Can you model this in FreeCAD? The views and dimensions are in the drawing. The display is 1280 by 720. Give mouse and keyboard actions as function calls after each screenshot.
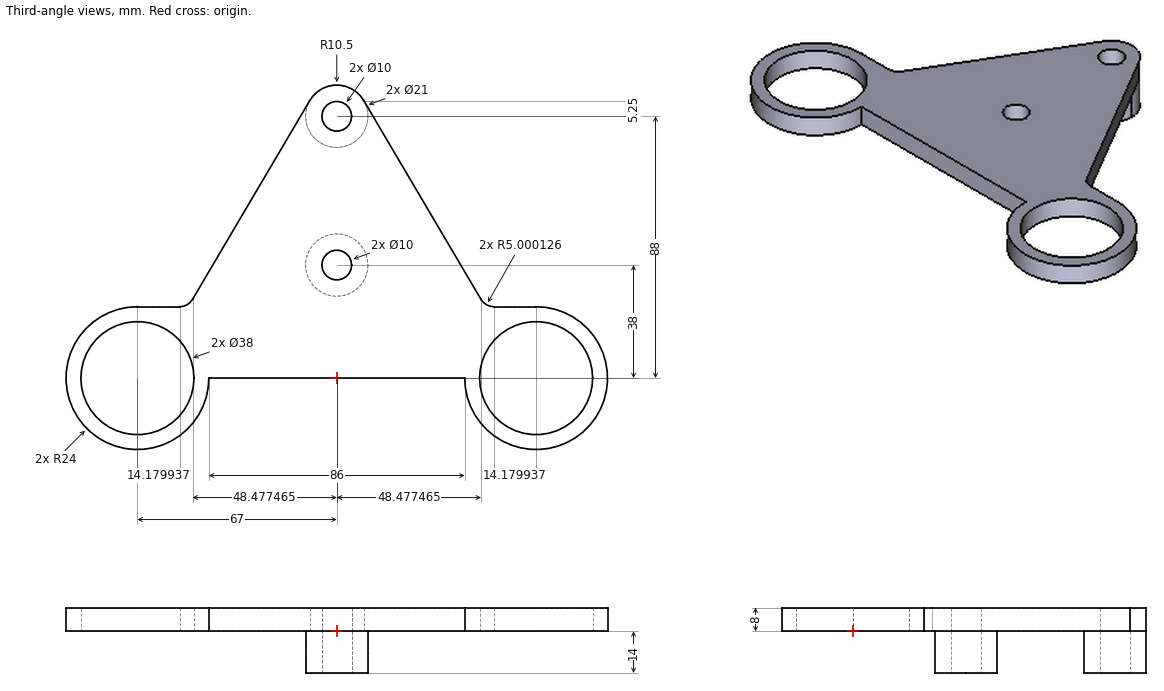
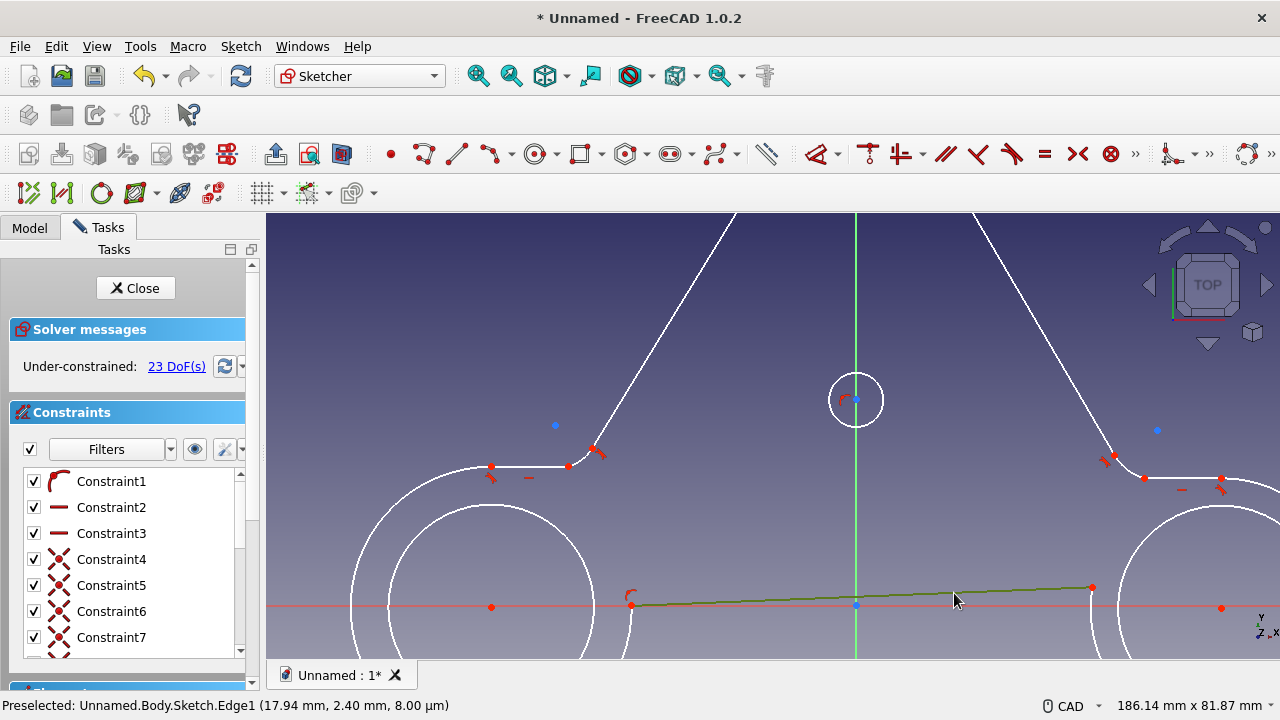
key(h)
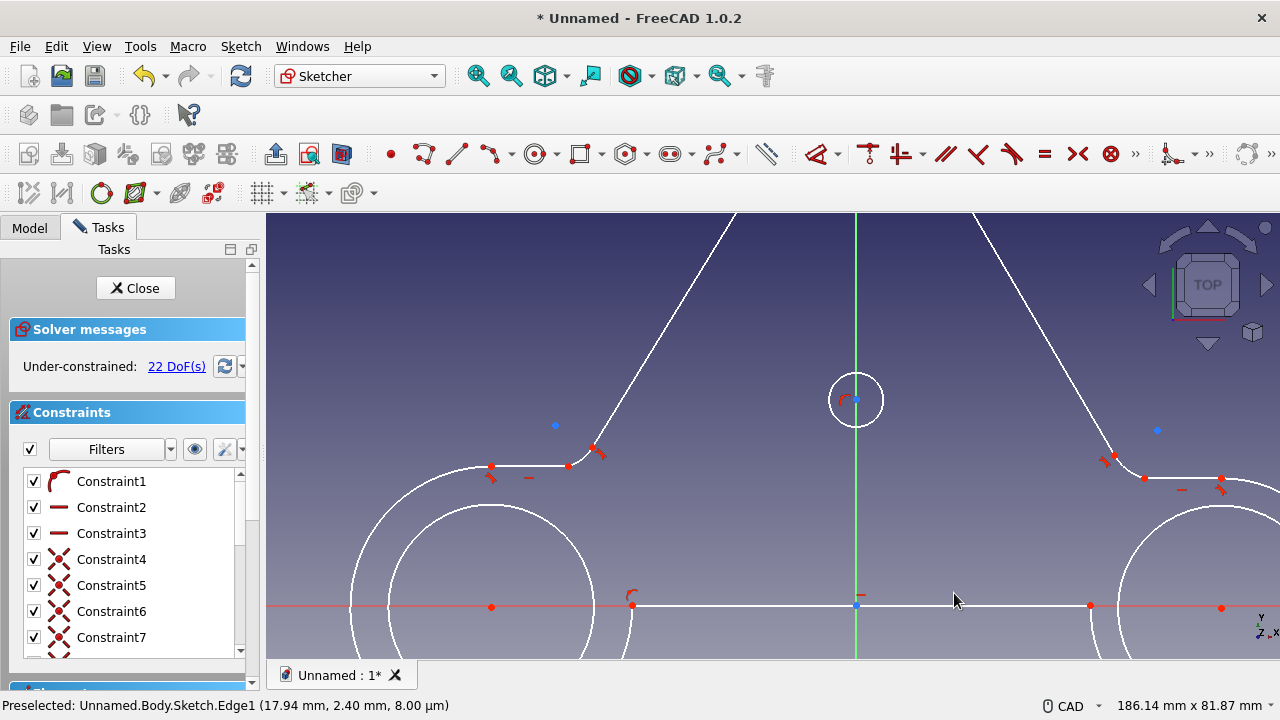
scroll(581, 474, down, 4)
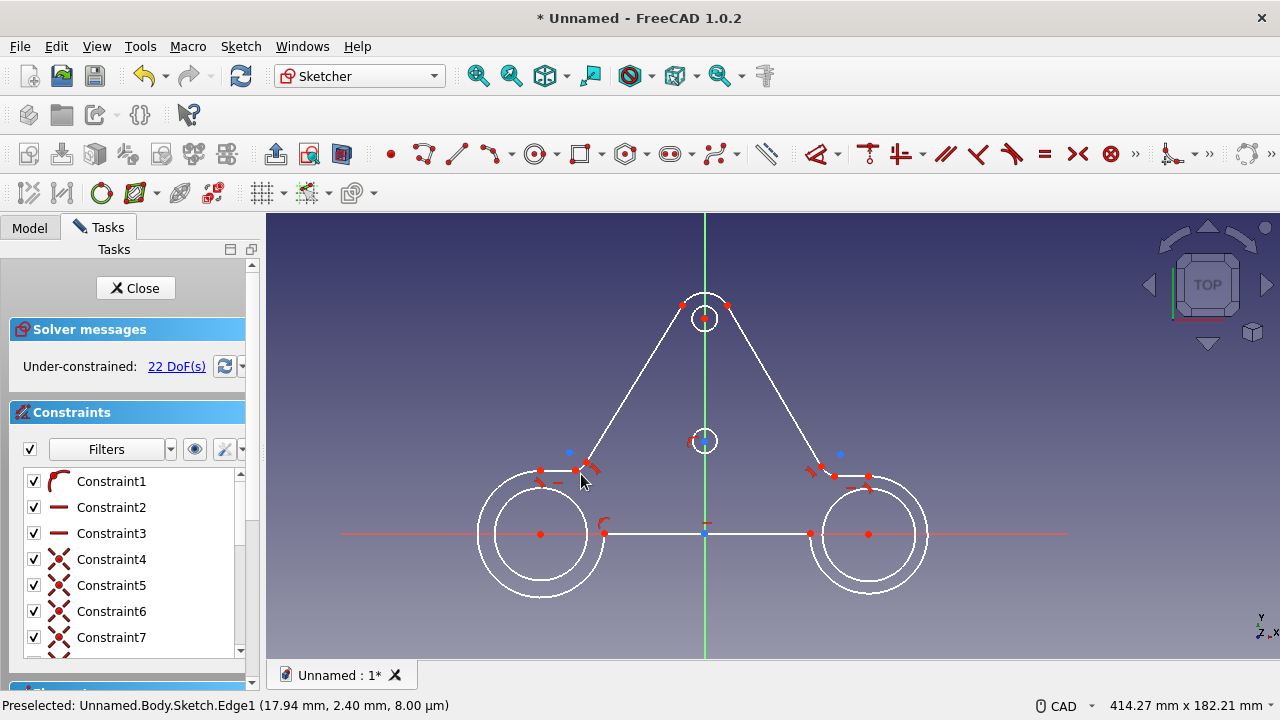
scroll(824, 470, up, 5)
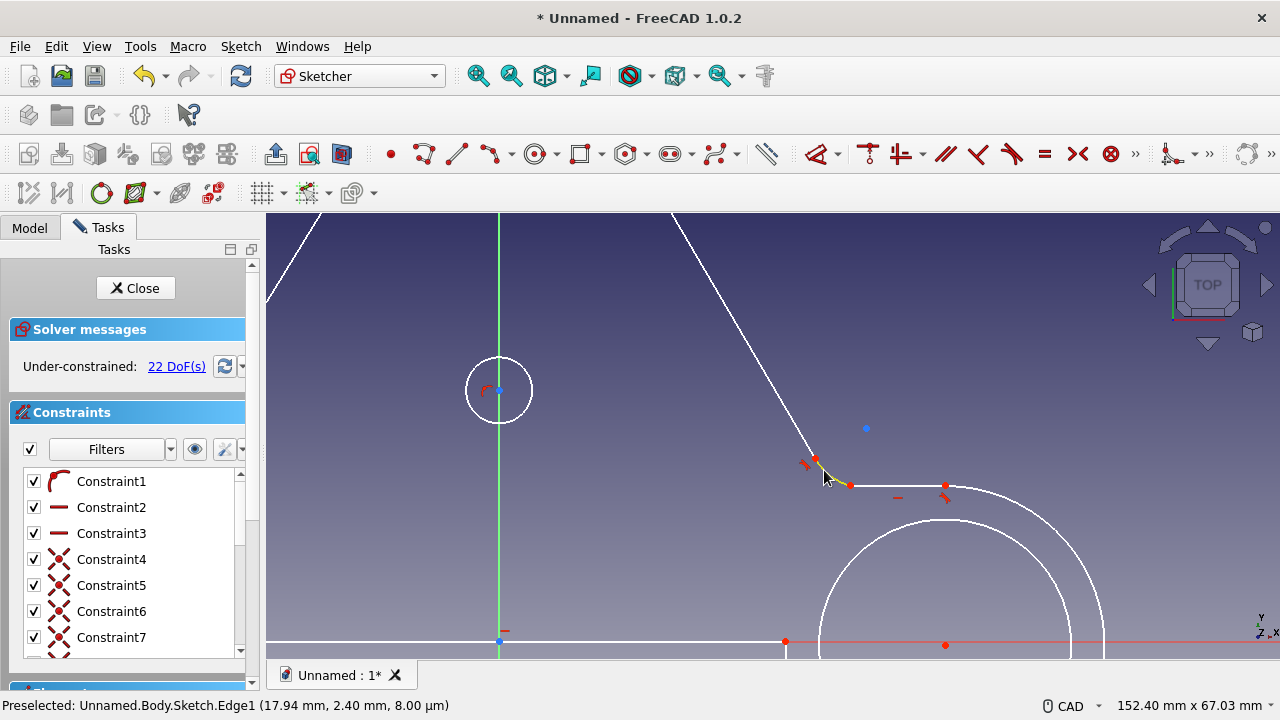
click(823, 470)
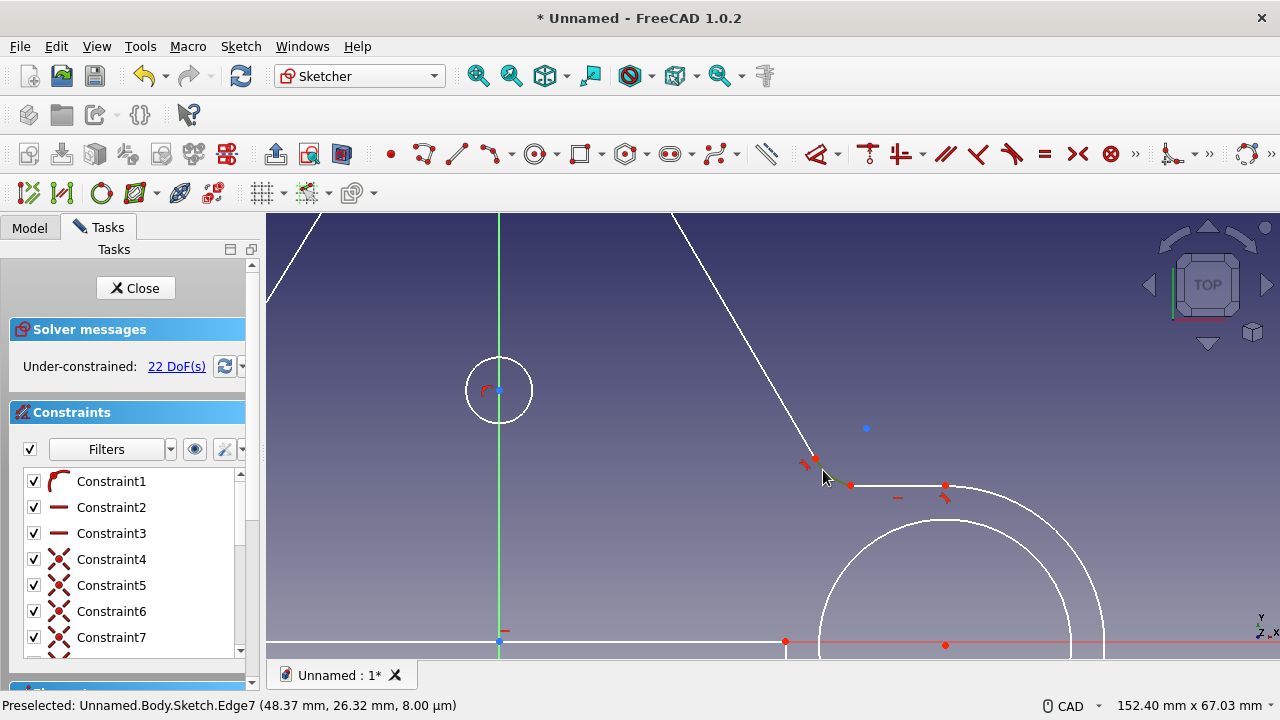
scroll(824, 470, down, 5)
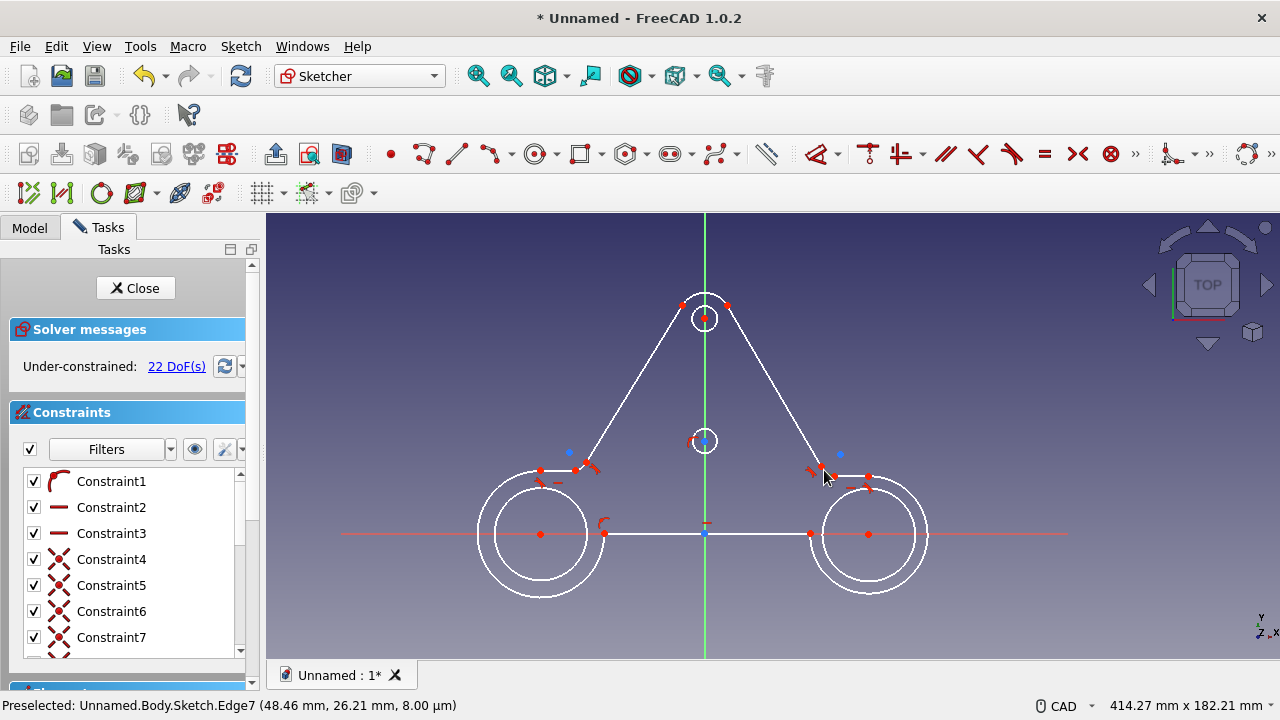
scroll(579, 469, up, 6)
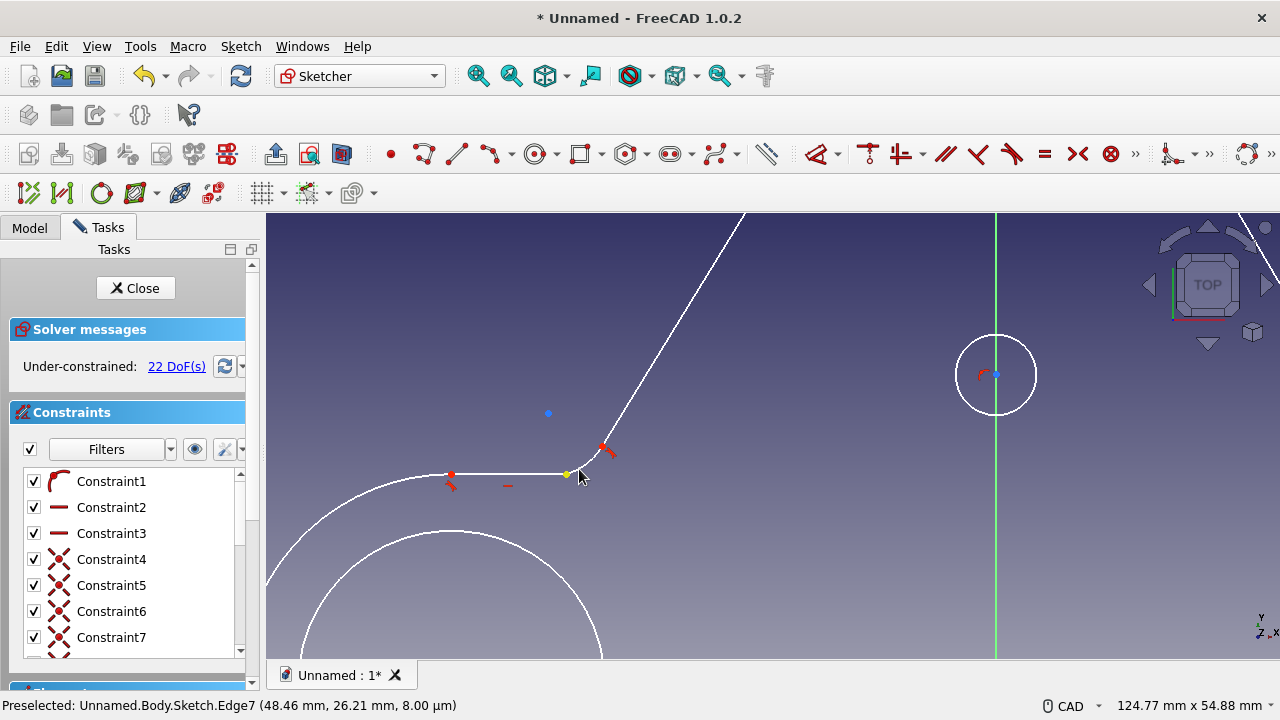
click(579, 469)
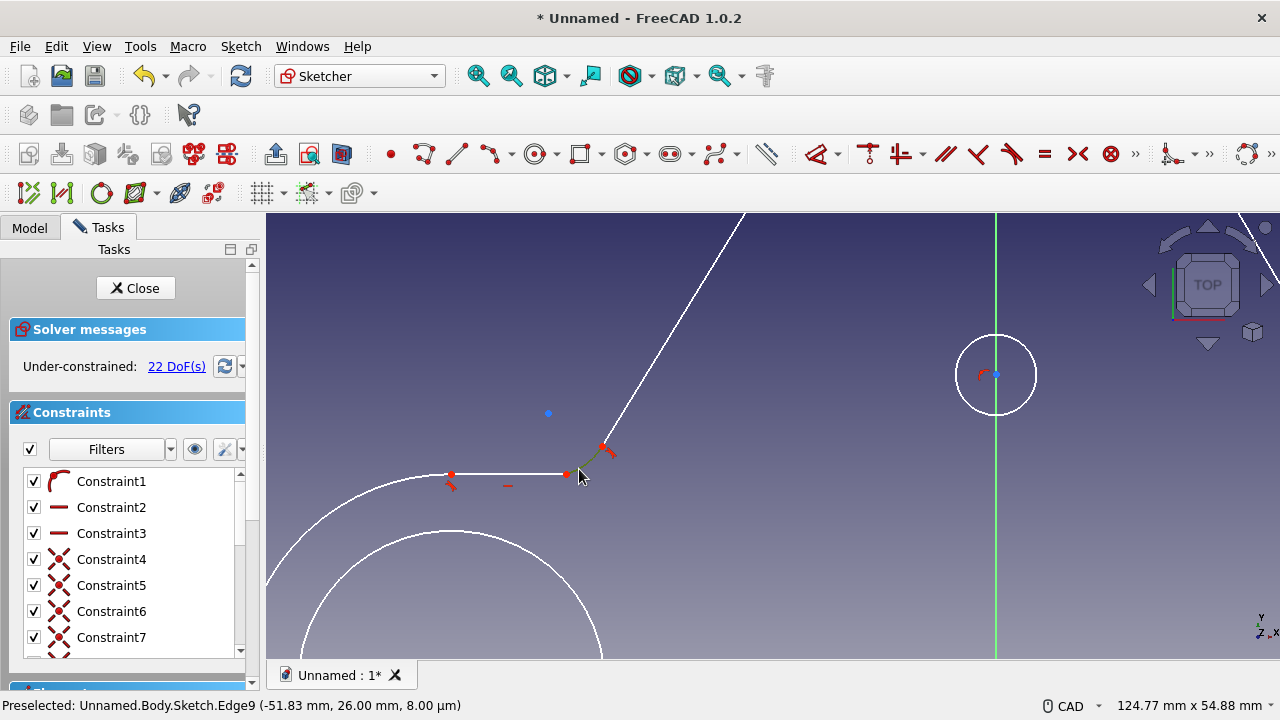
key(e)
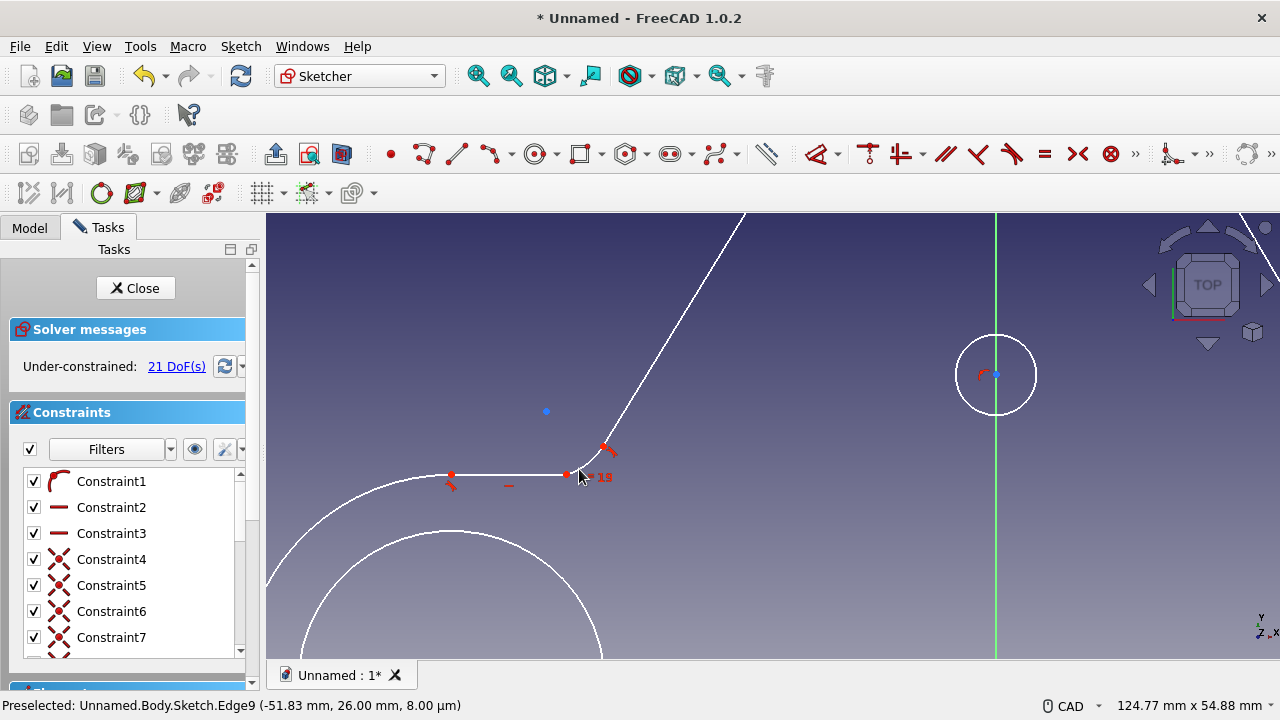
scroll(579, 469, down, 6)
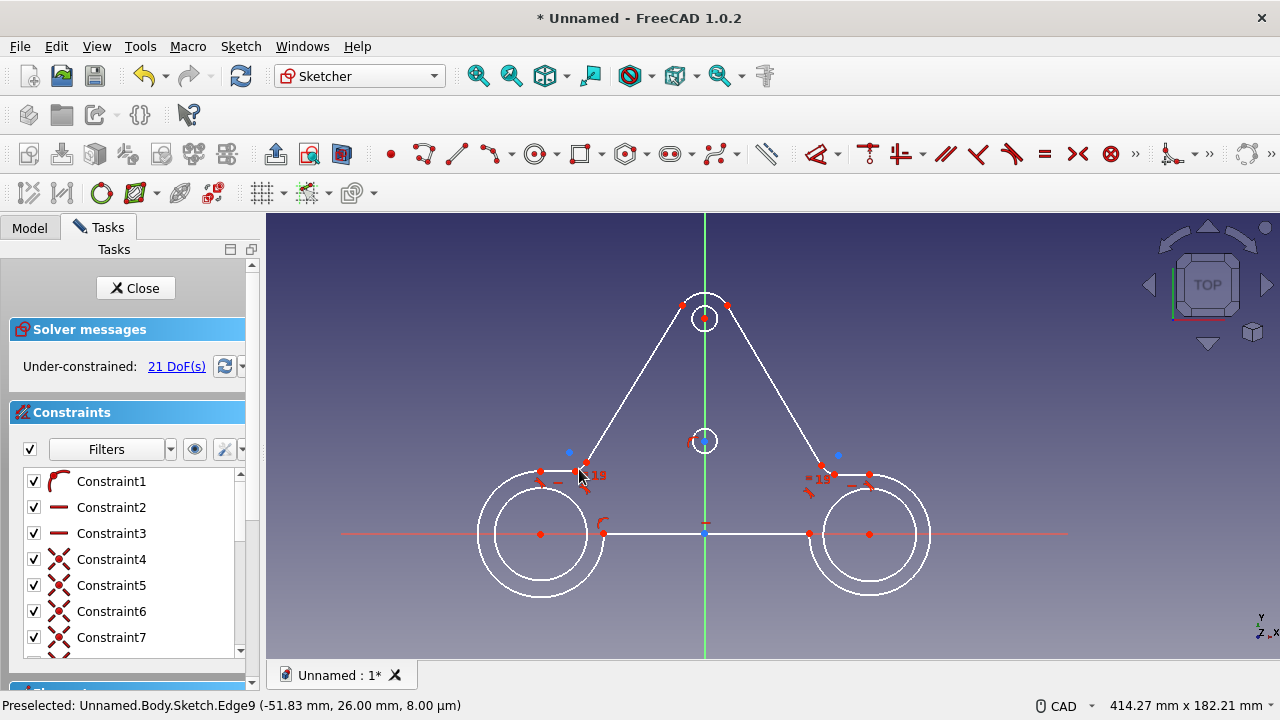
click(859, 594)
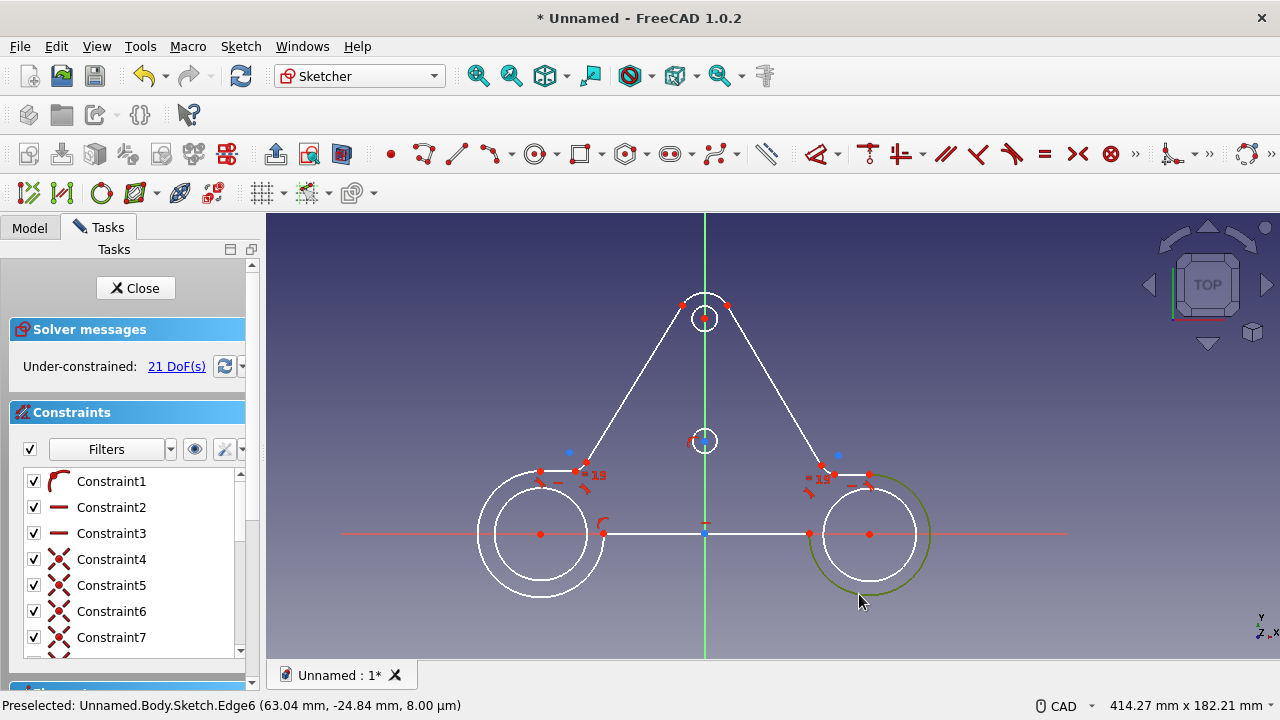
scroll(478, 525, up, 3)